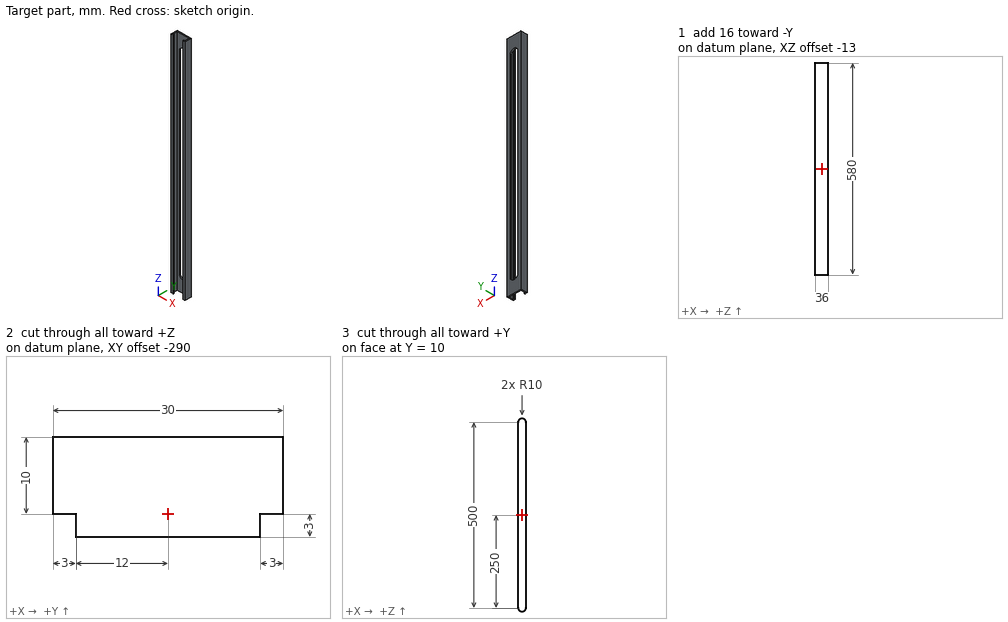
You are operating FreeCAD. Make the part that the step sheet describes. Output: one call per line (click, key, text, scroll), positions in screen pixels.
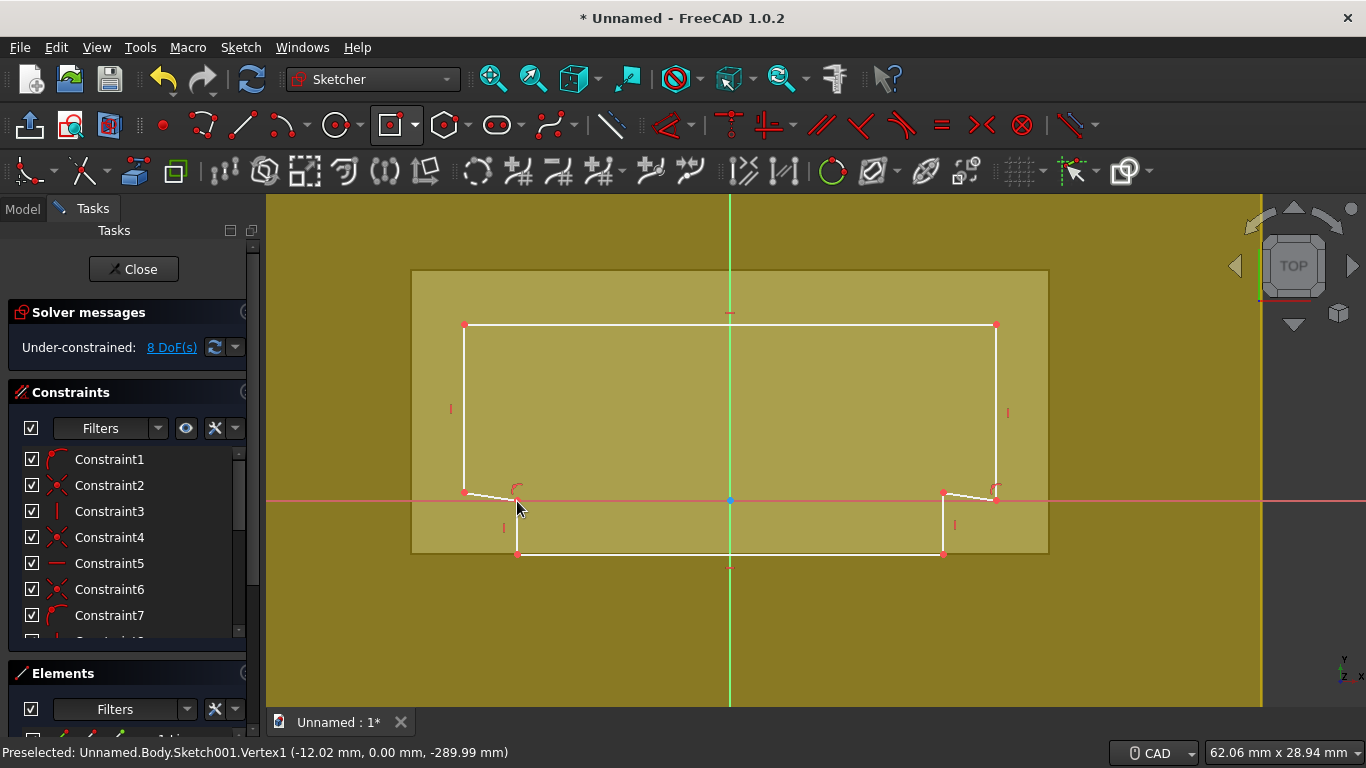
click(501, 499)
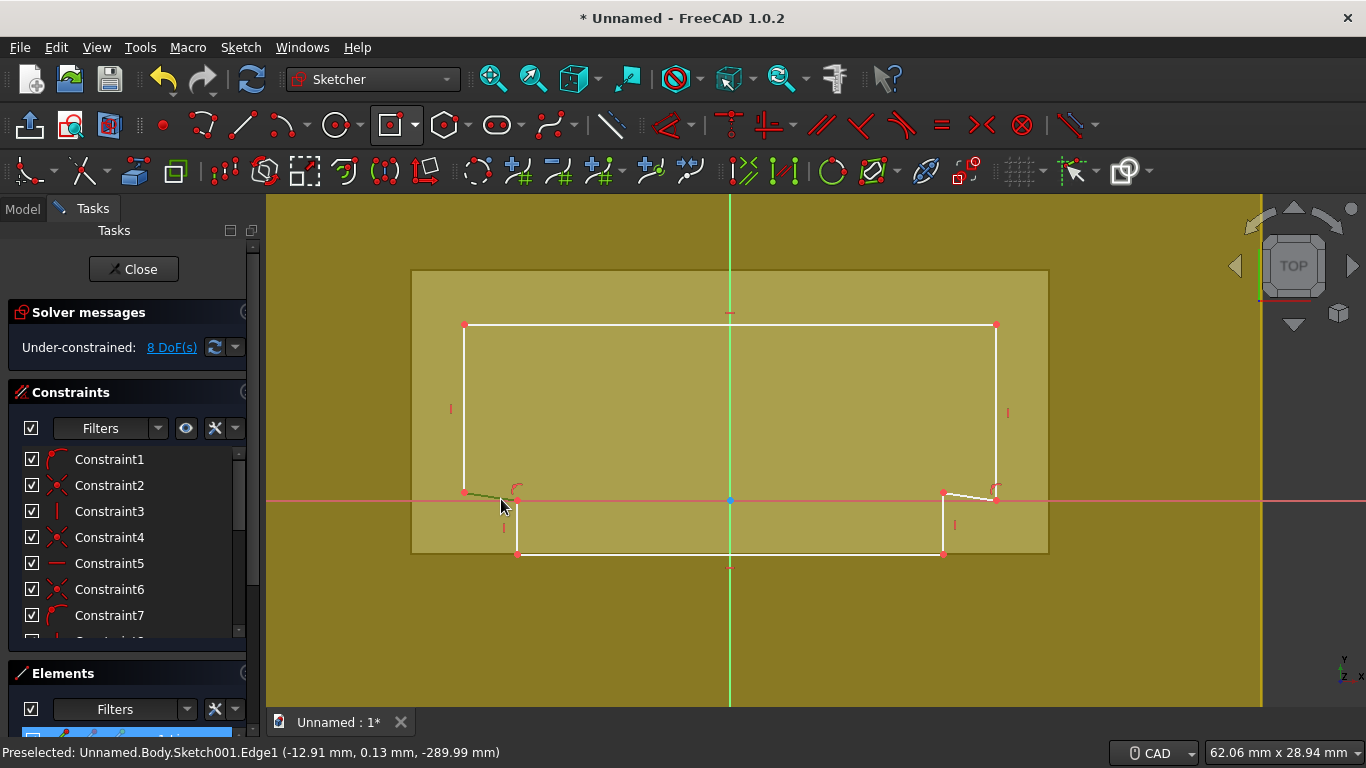
click(796, 126)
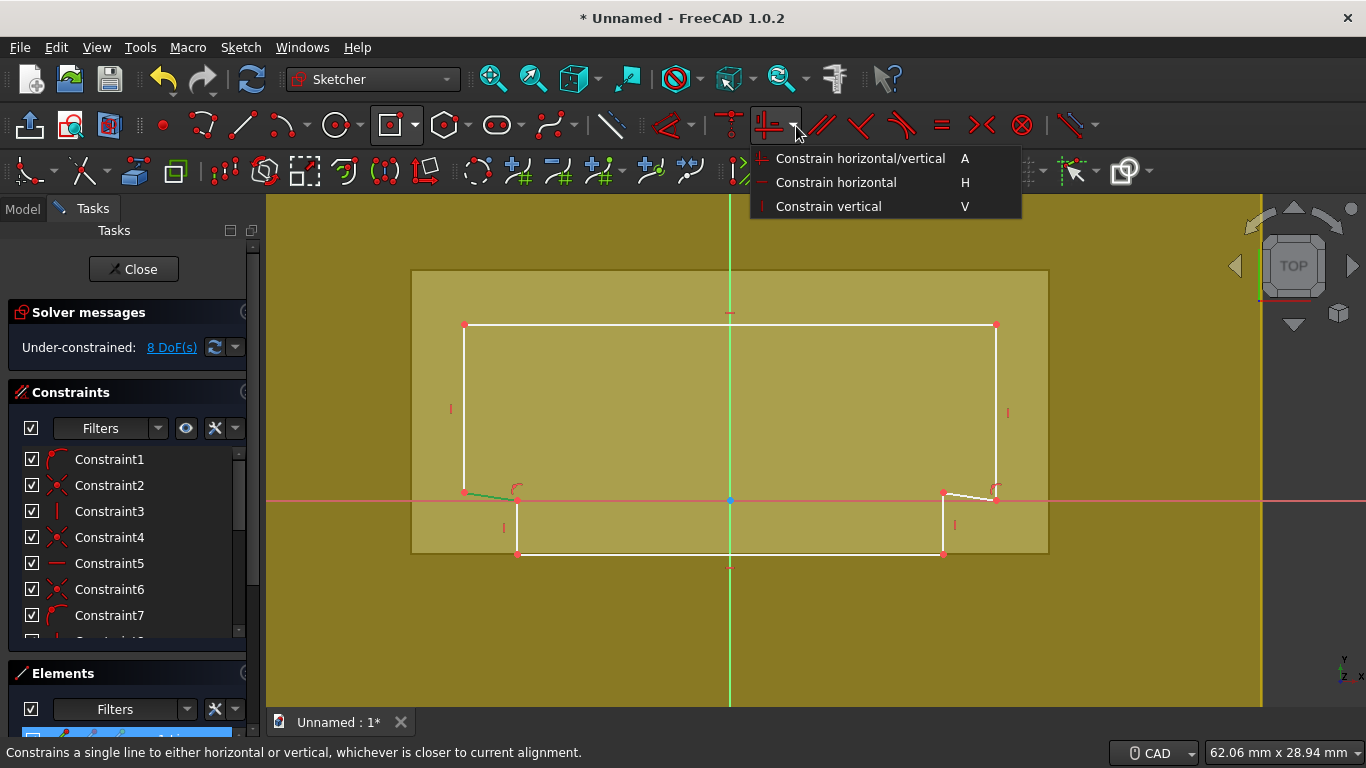
click(886, 182)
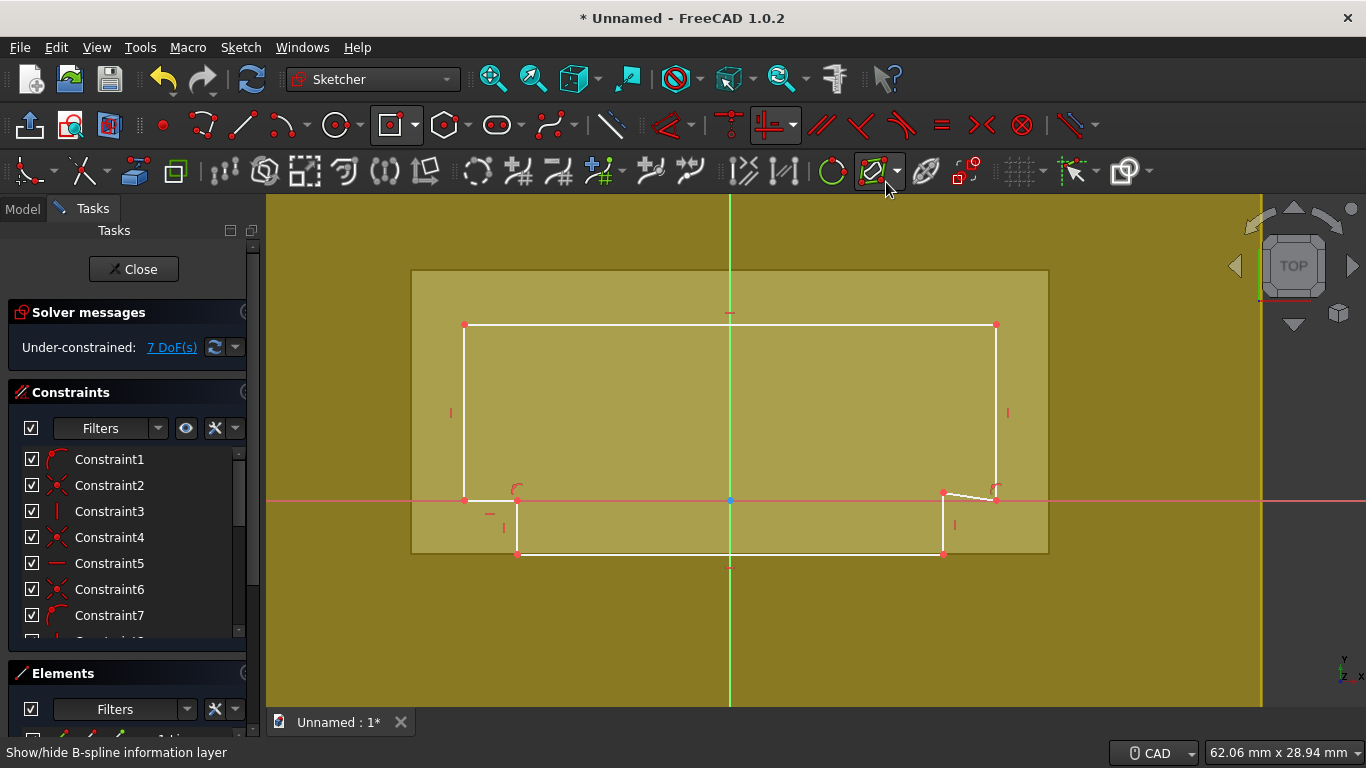
click(980, 499)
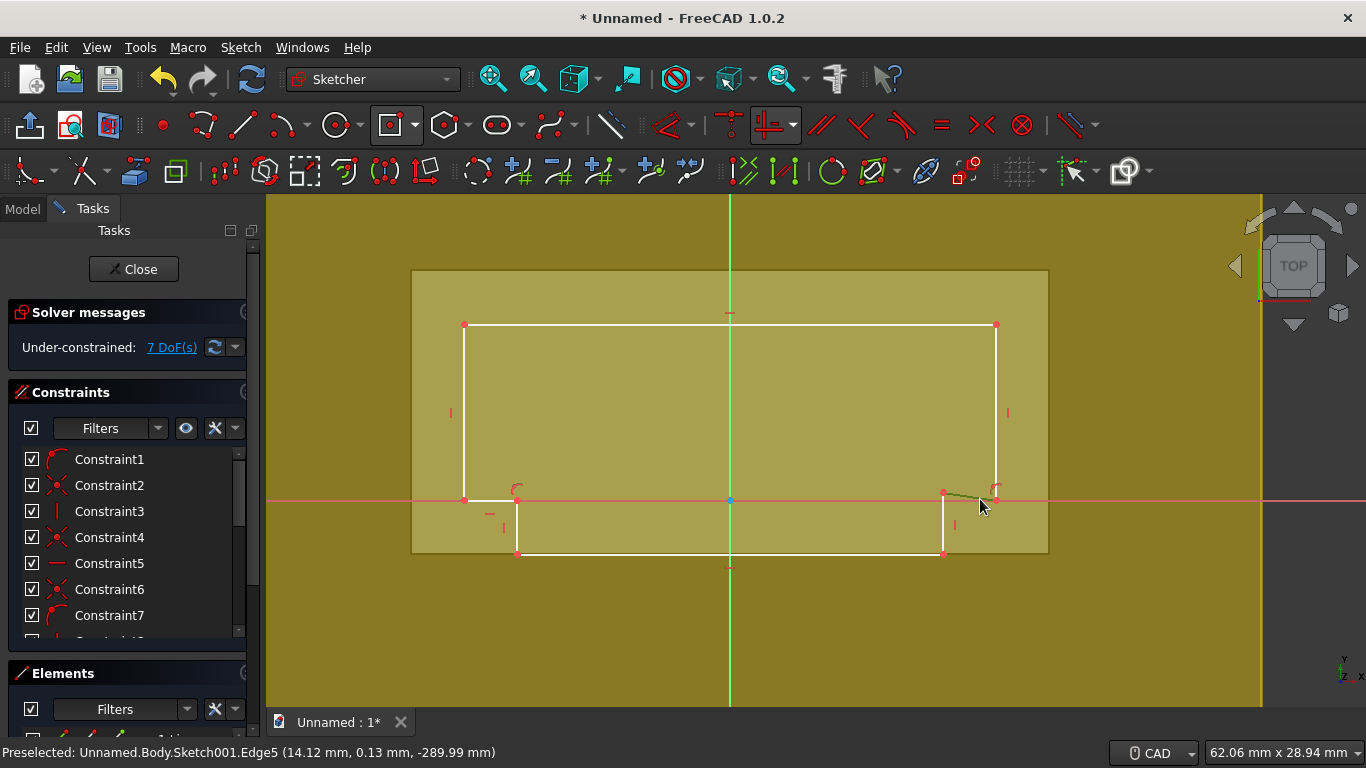
click(796, 126)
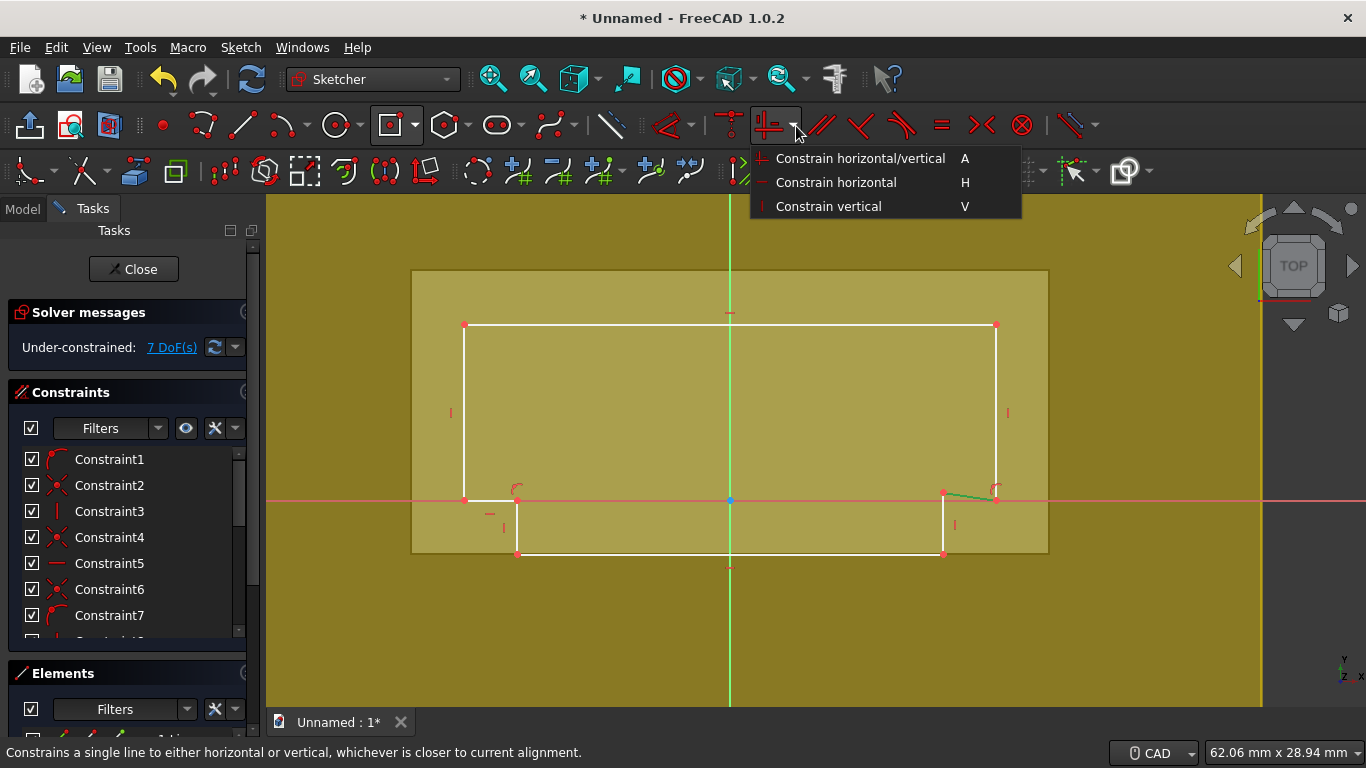
click(886, 182)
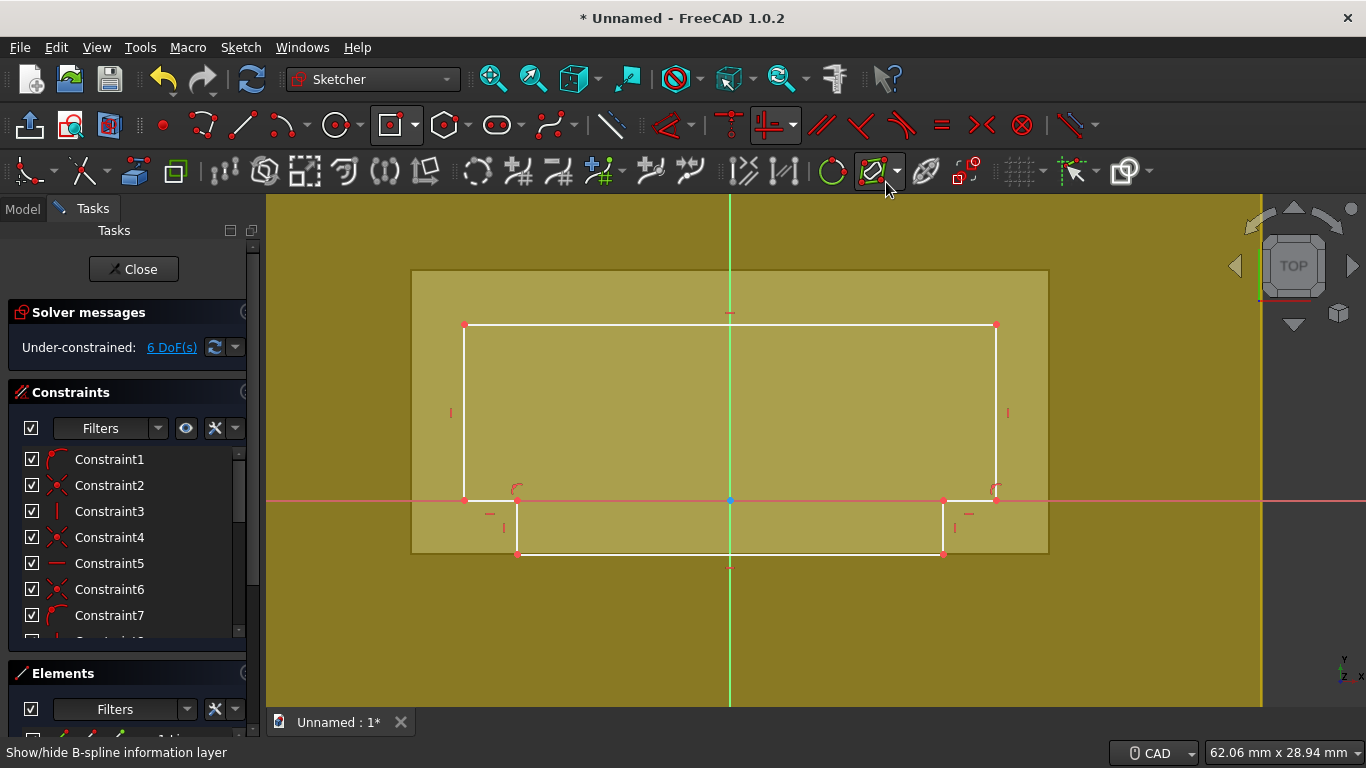
click(666, 126)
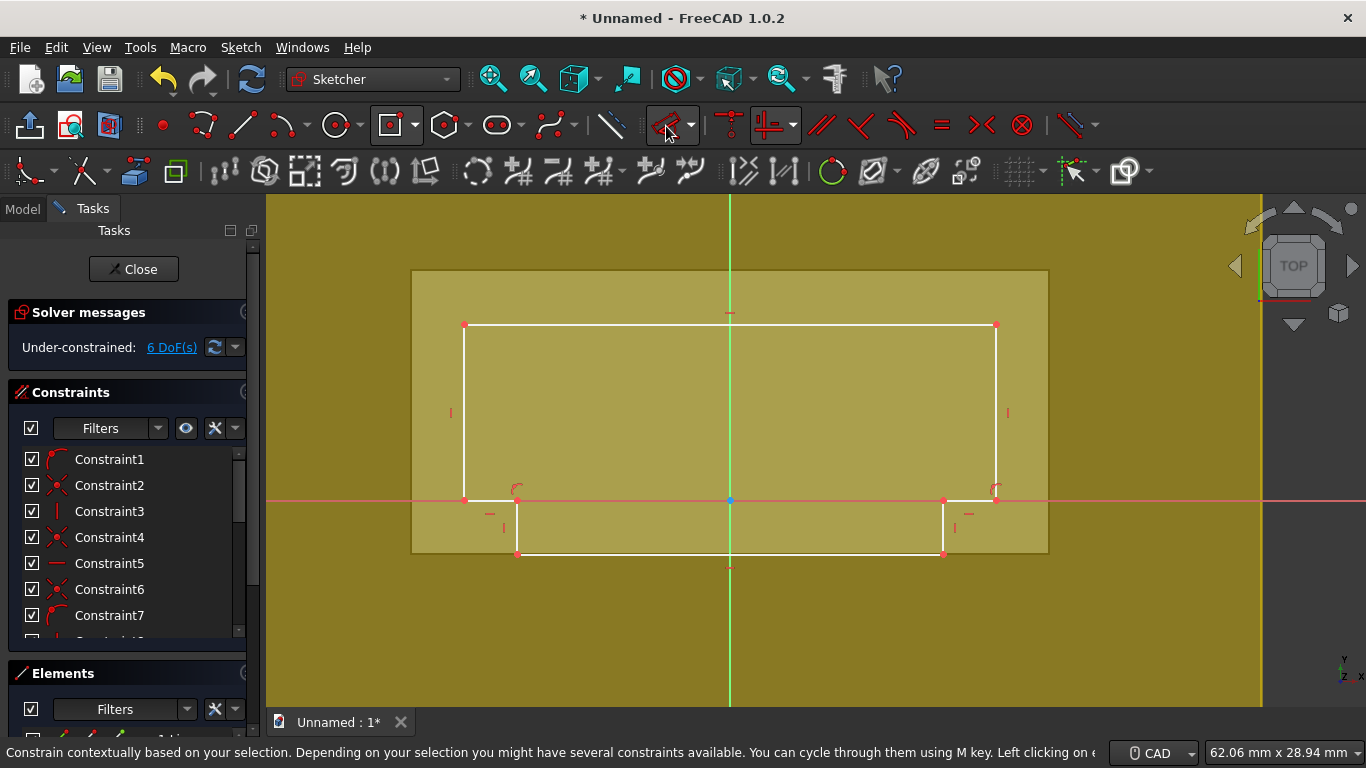
click(501, 501)
click(491, 535)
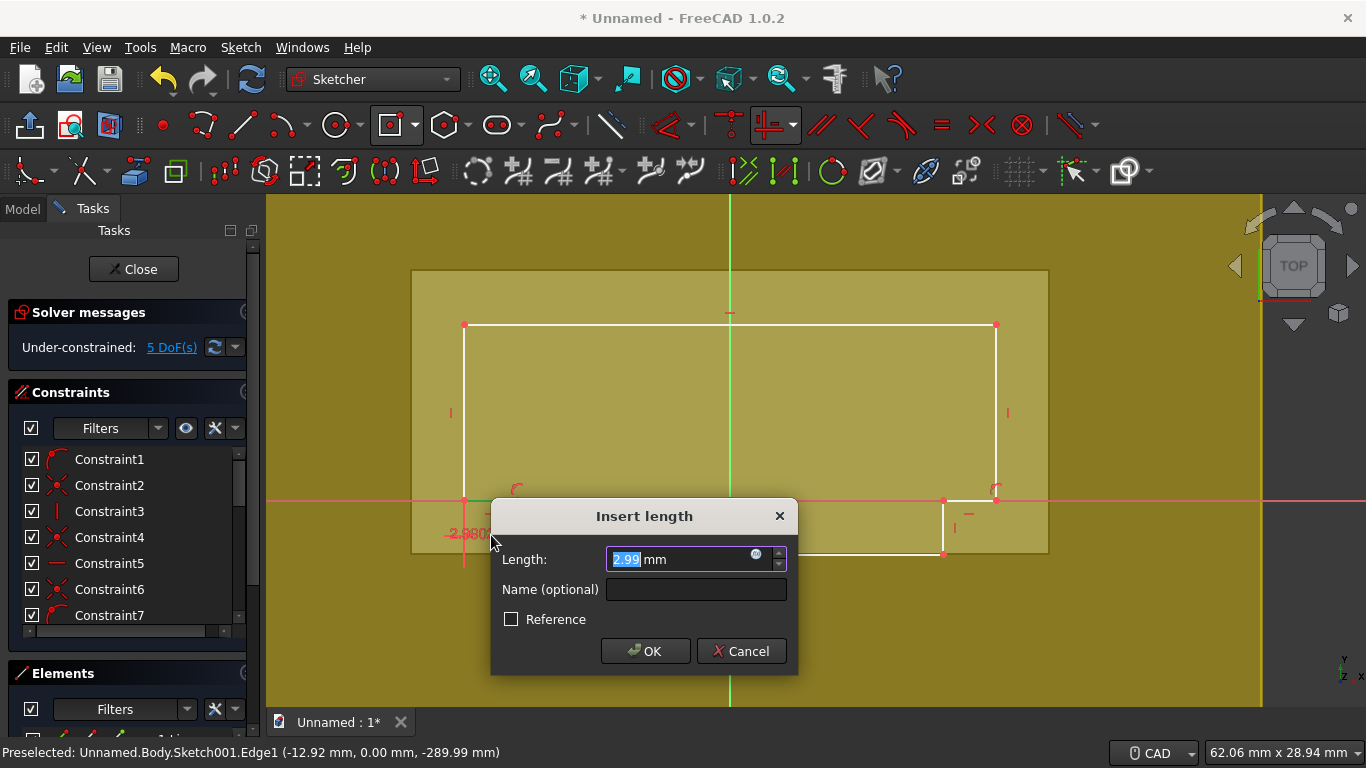
text(3)
key(Return)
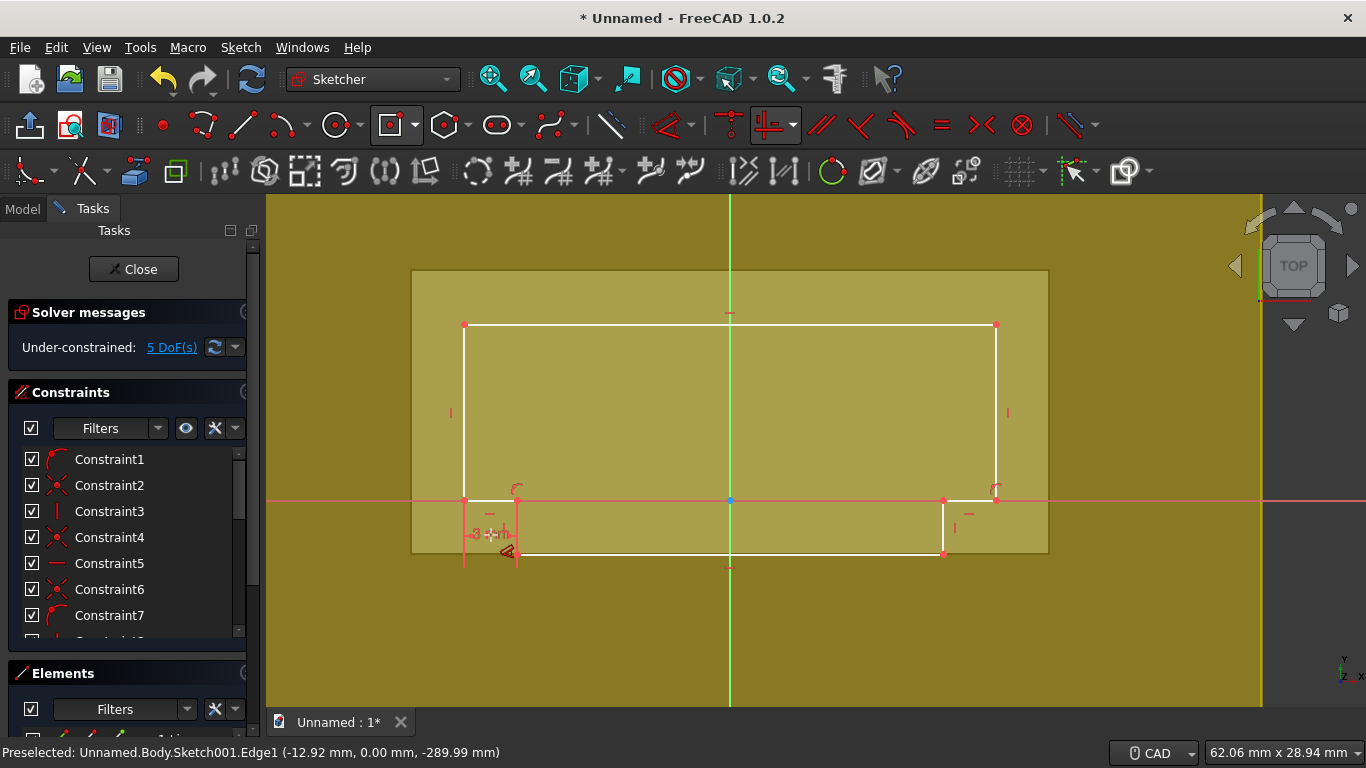
click(980, 501)
click(970, 535)